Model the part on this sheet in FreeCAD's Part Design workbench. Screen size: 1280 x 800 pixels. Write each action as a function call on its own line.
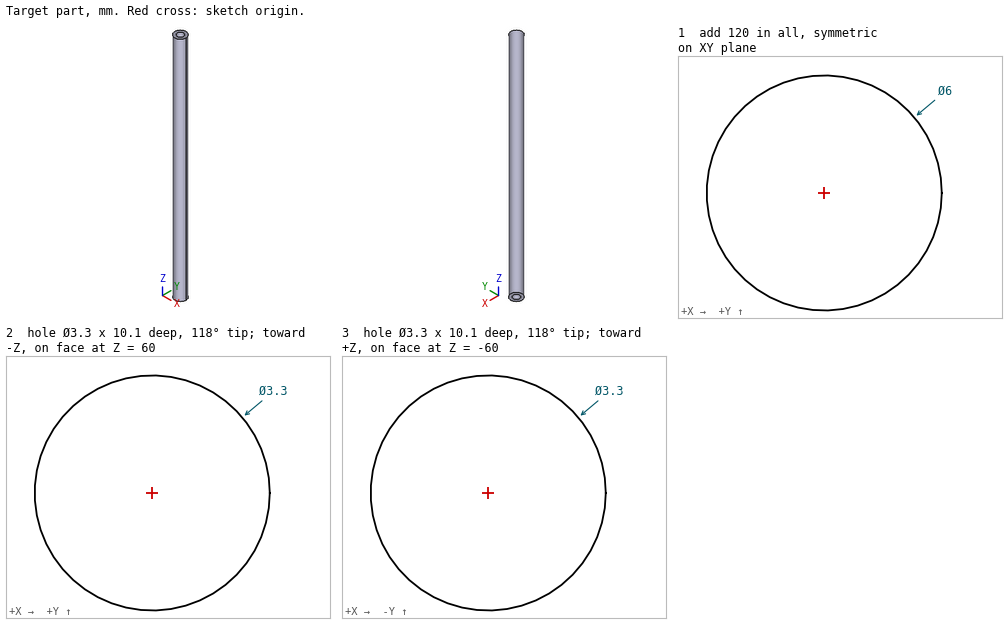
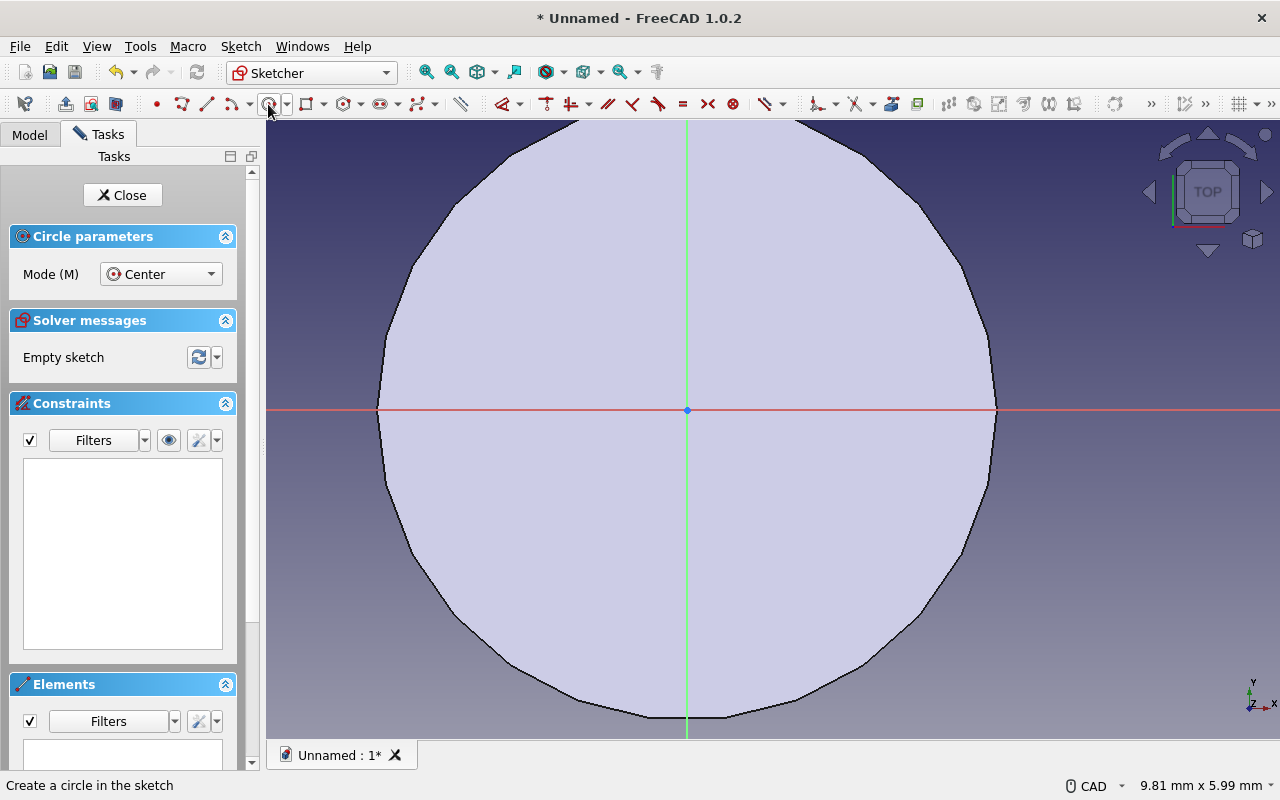
click(687, 410)
click(808, 290)
key(Escape)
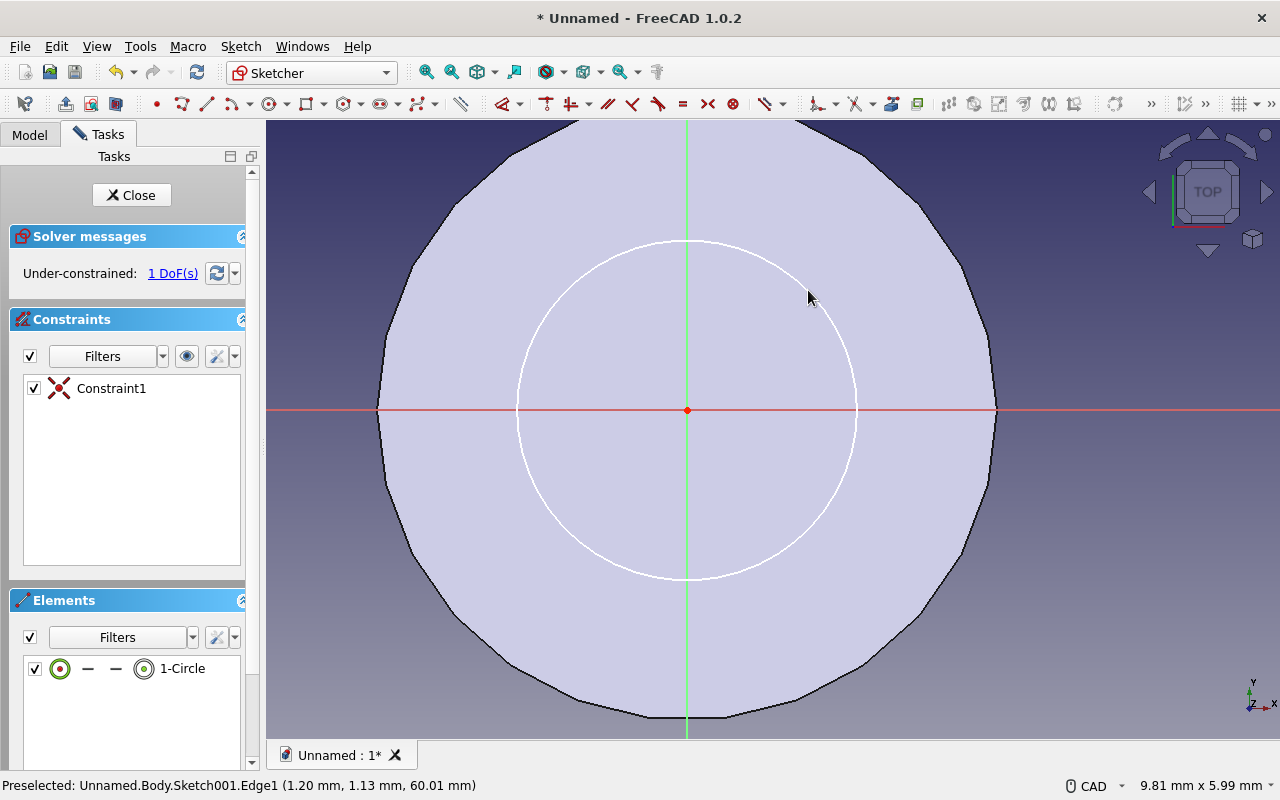
click(502, 104)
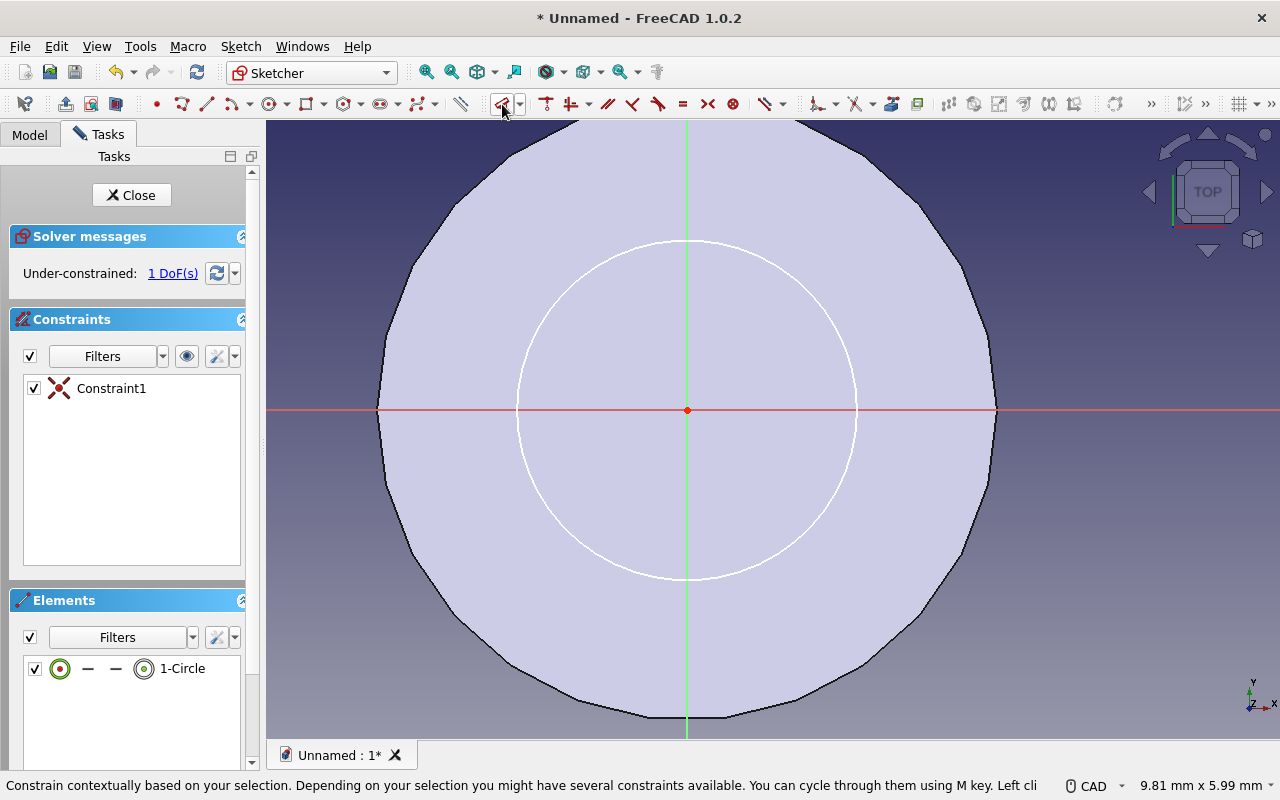
click(807, 290)
click(830, 267)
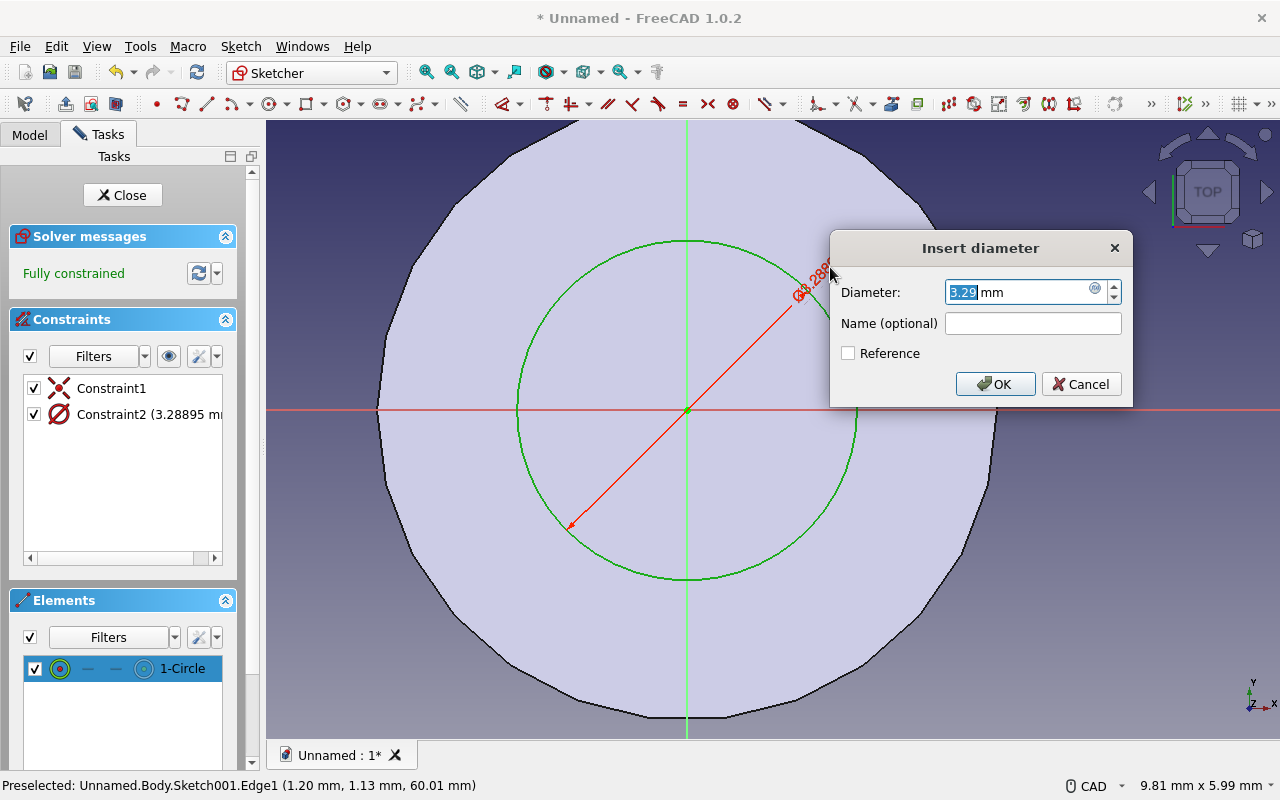
text(3.3)
key(Return)
key(Escape)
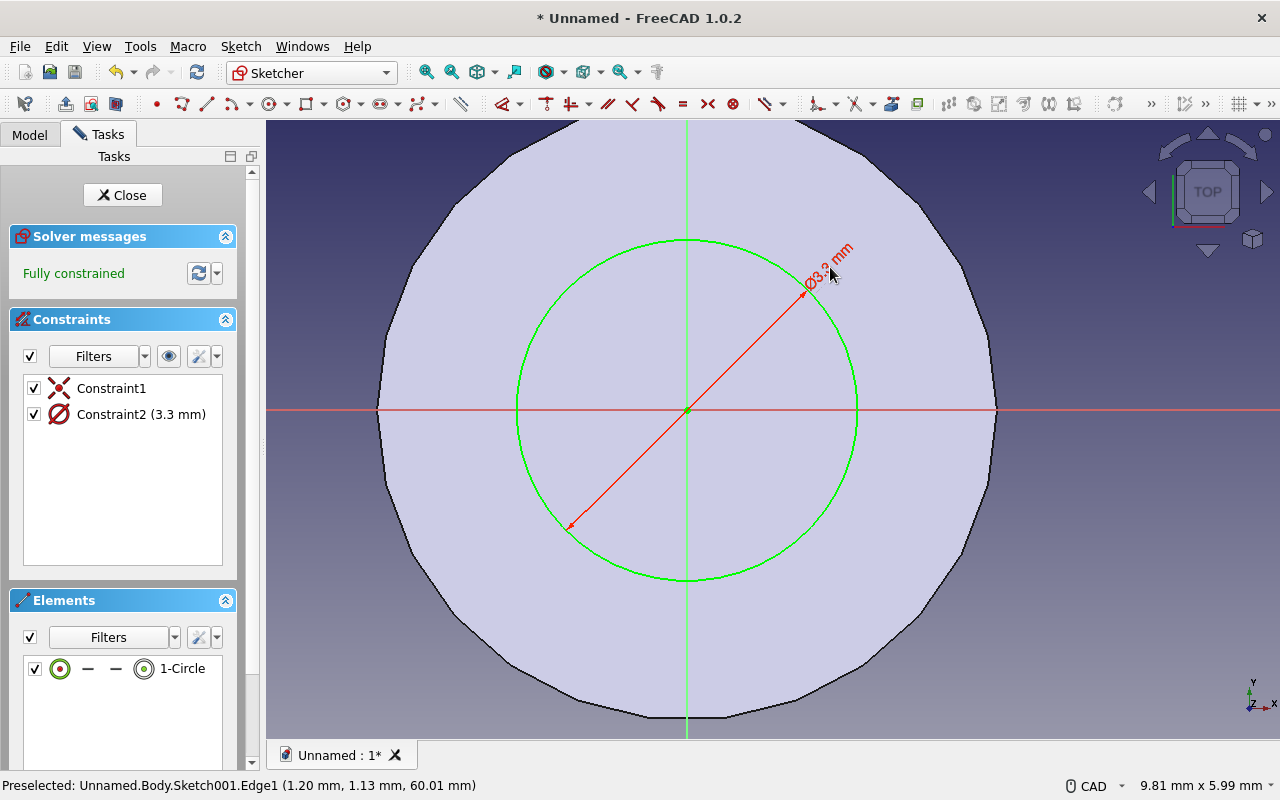
click(123, 195)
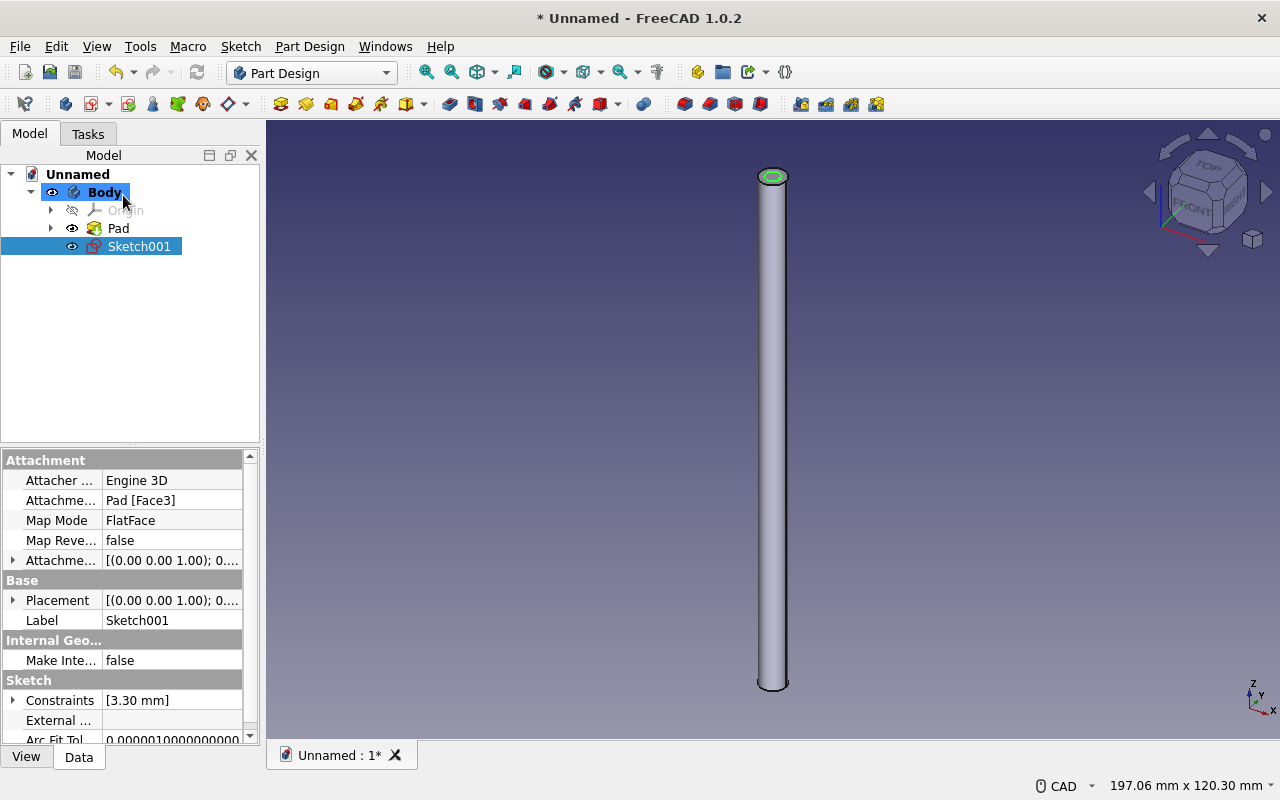
click(475, 104)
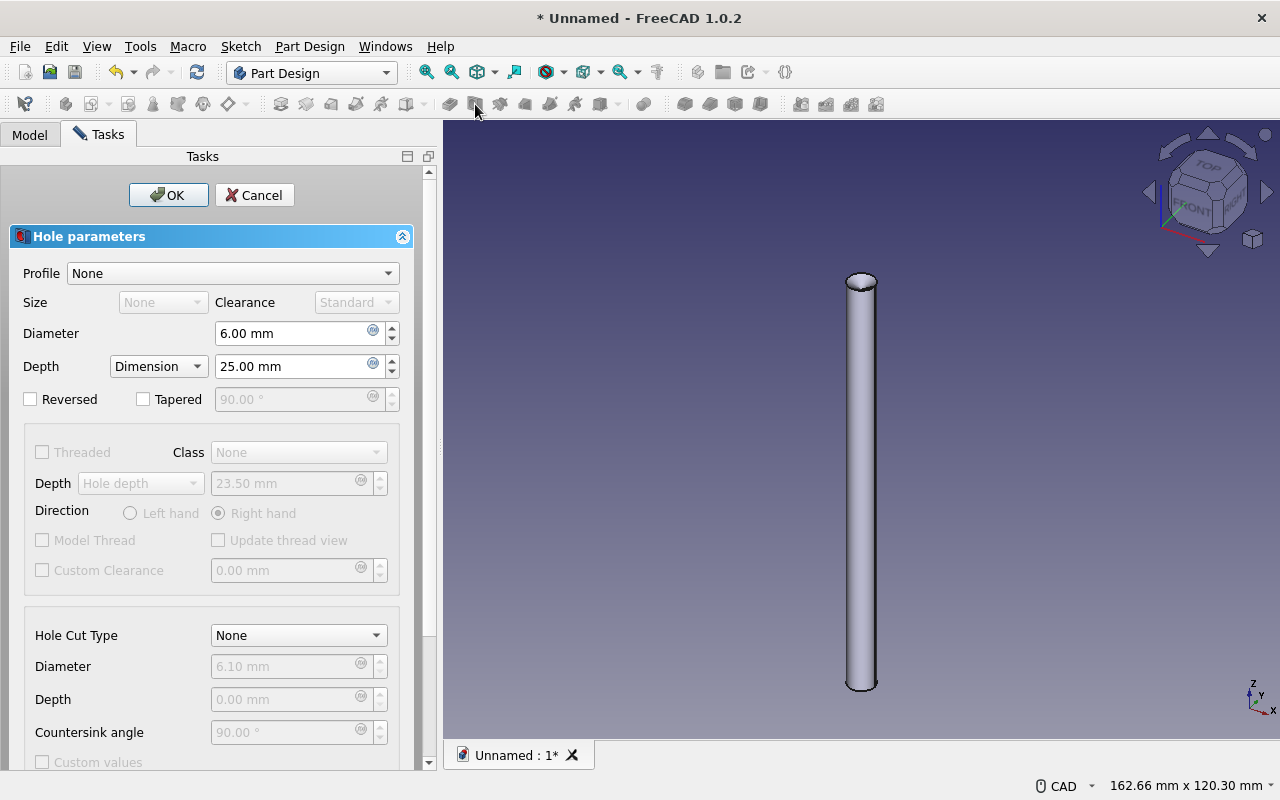
triple_click(300, 334)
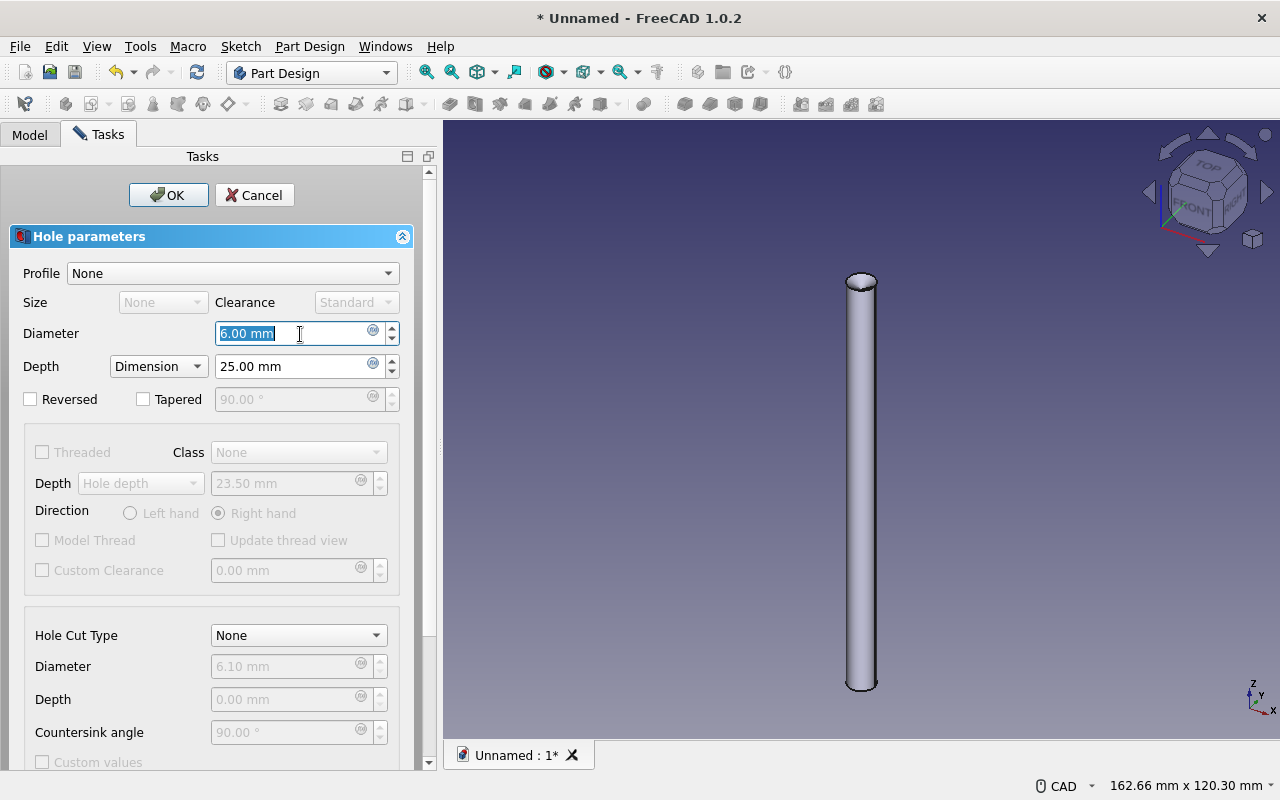
text(3.3)
key(Tab)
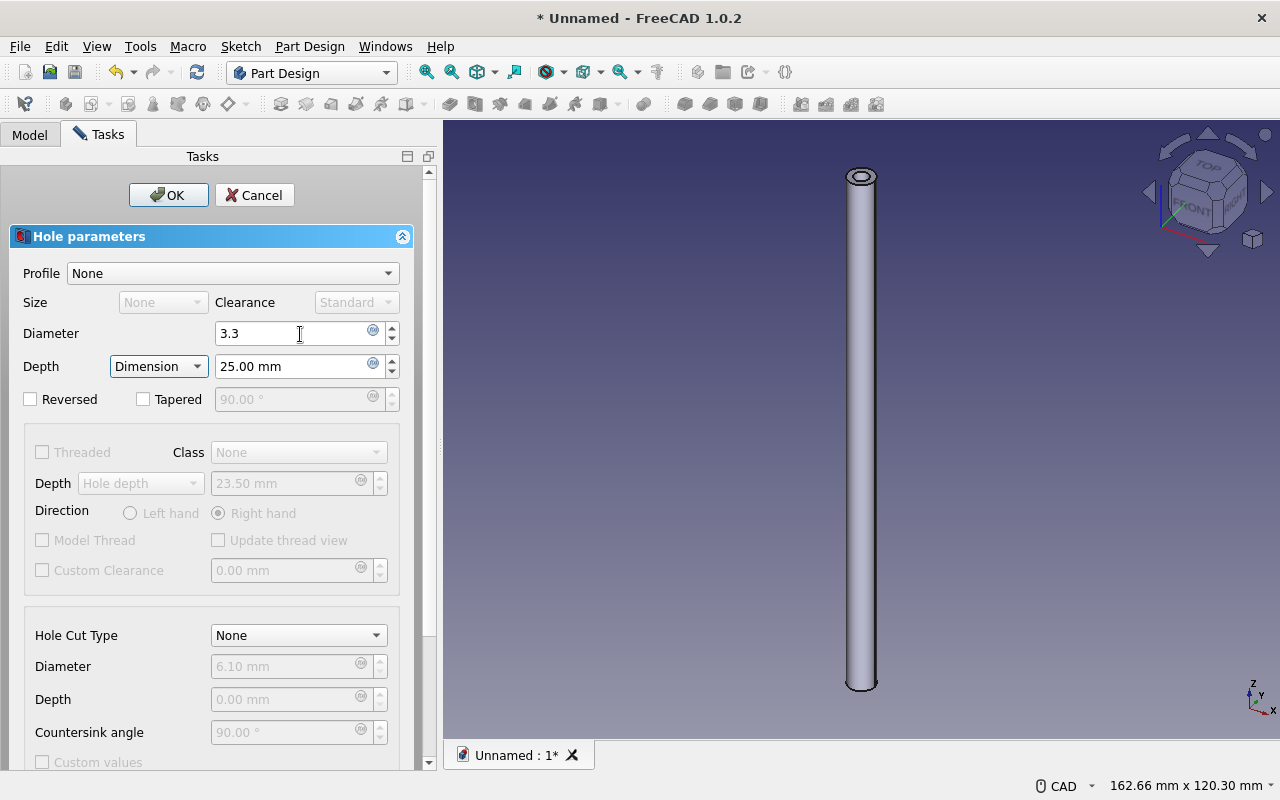
triple_click(300, 366)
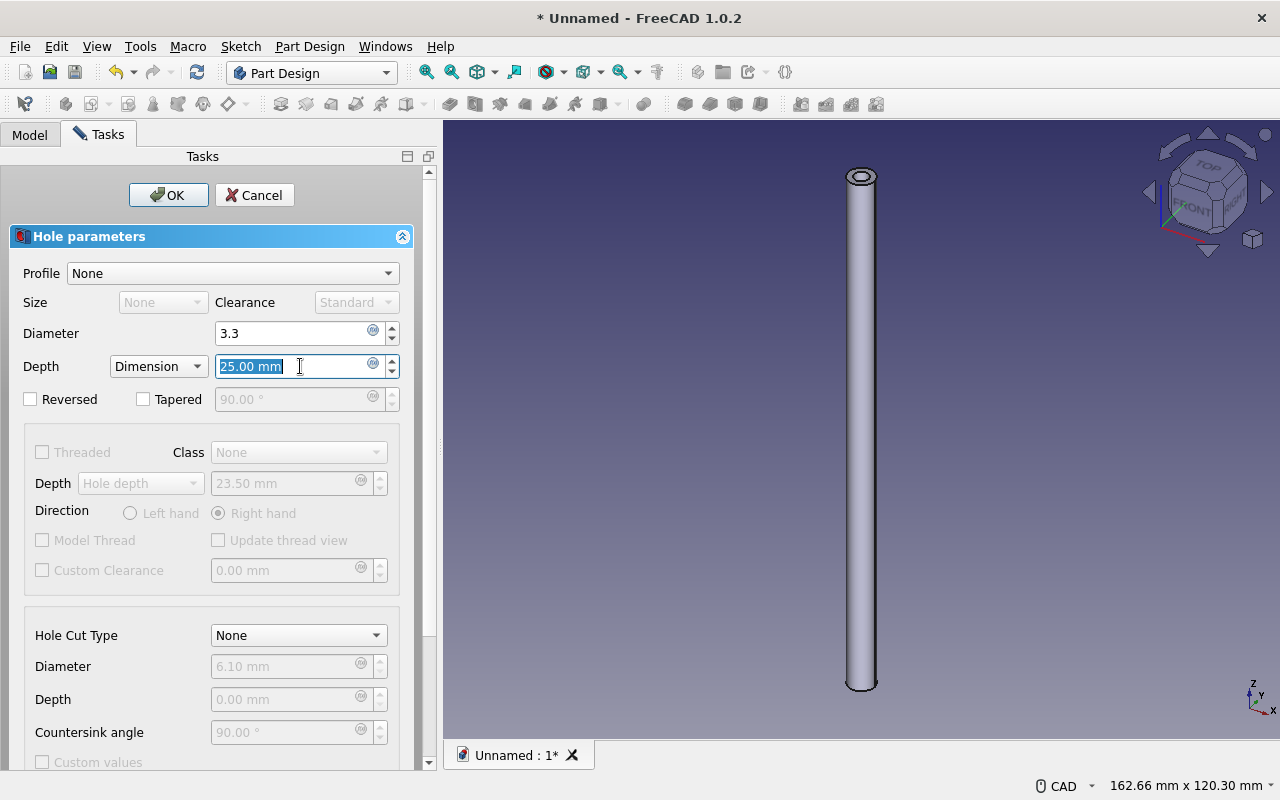
text(10.1)
key(Tab)